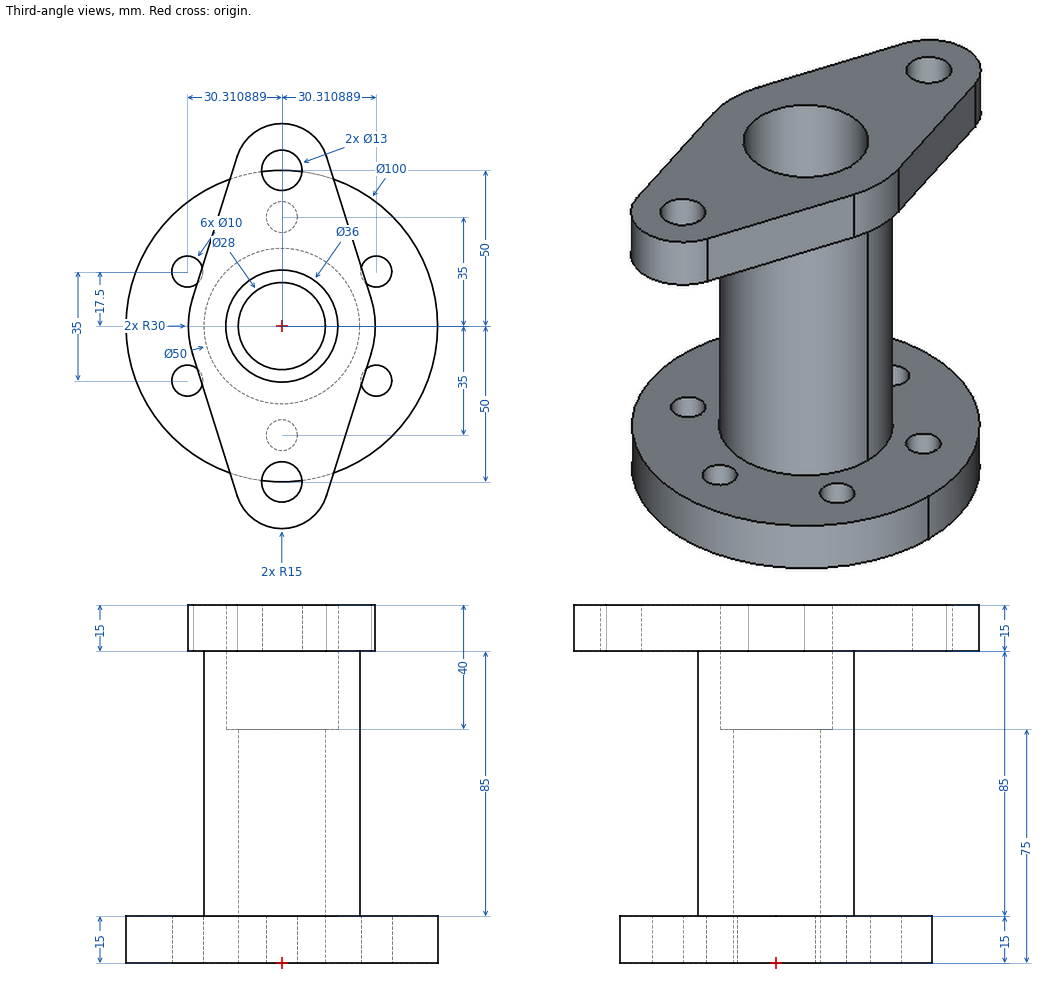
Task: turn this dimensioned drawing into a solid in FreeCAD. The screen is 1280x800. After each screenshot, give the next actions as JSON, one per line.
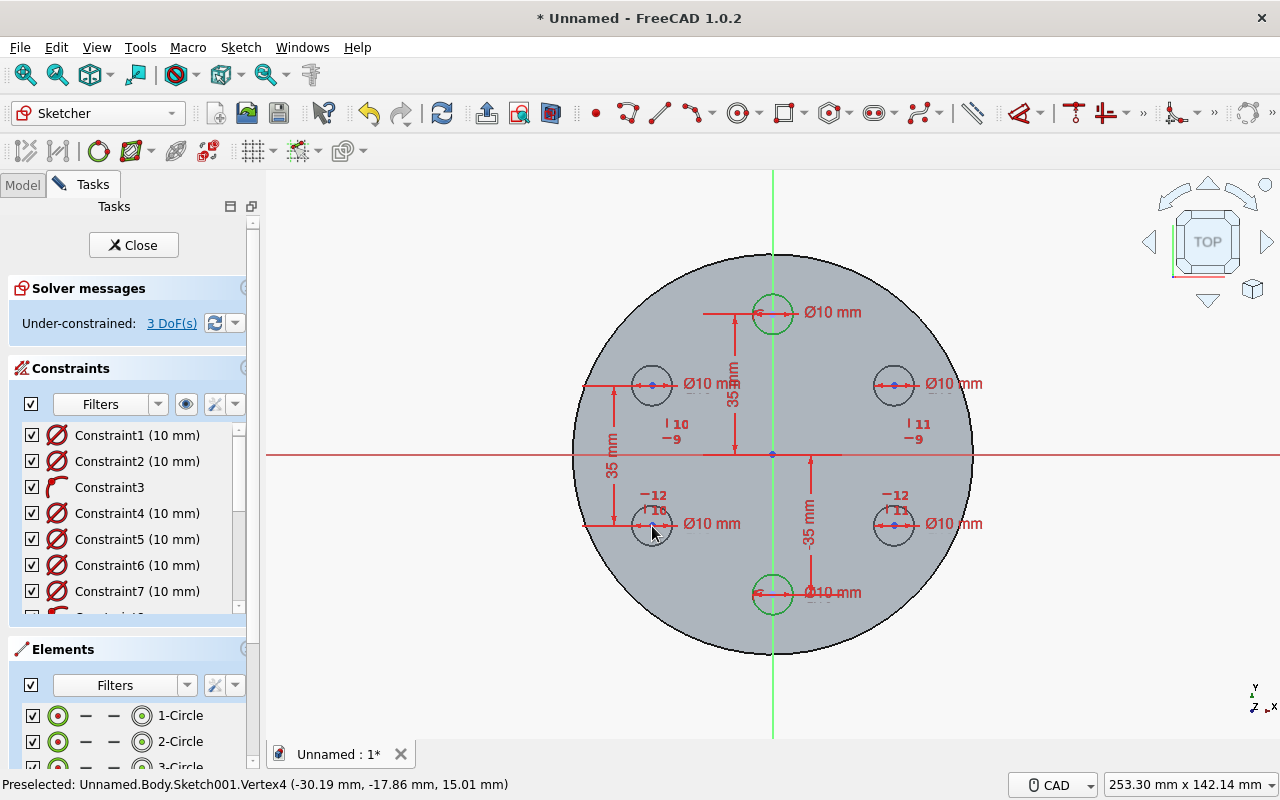
{"action": "left_click", "coordinate": [652, 386]}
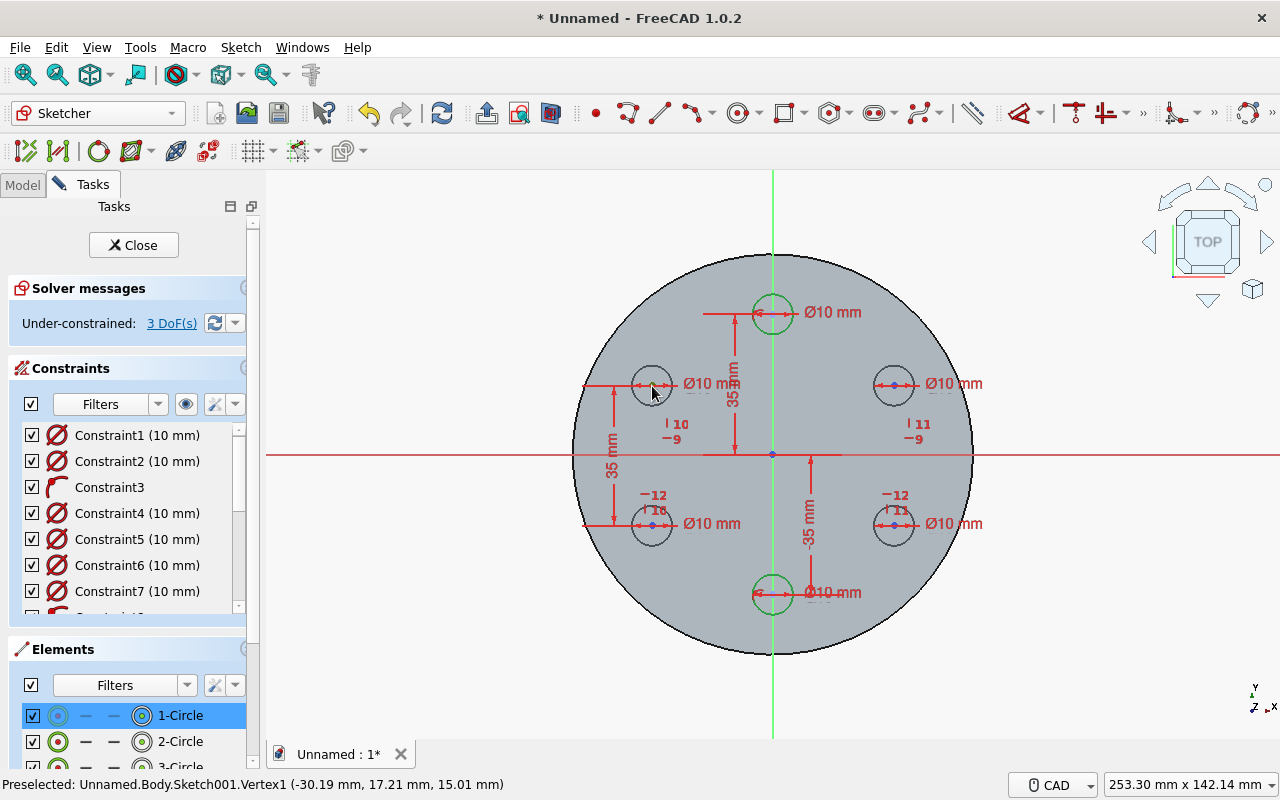
{"action": "key", "text": "i"}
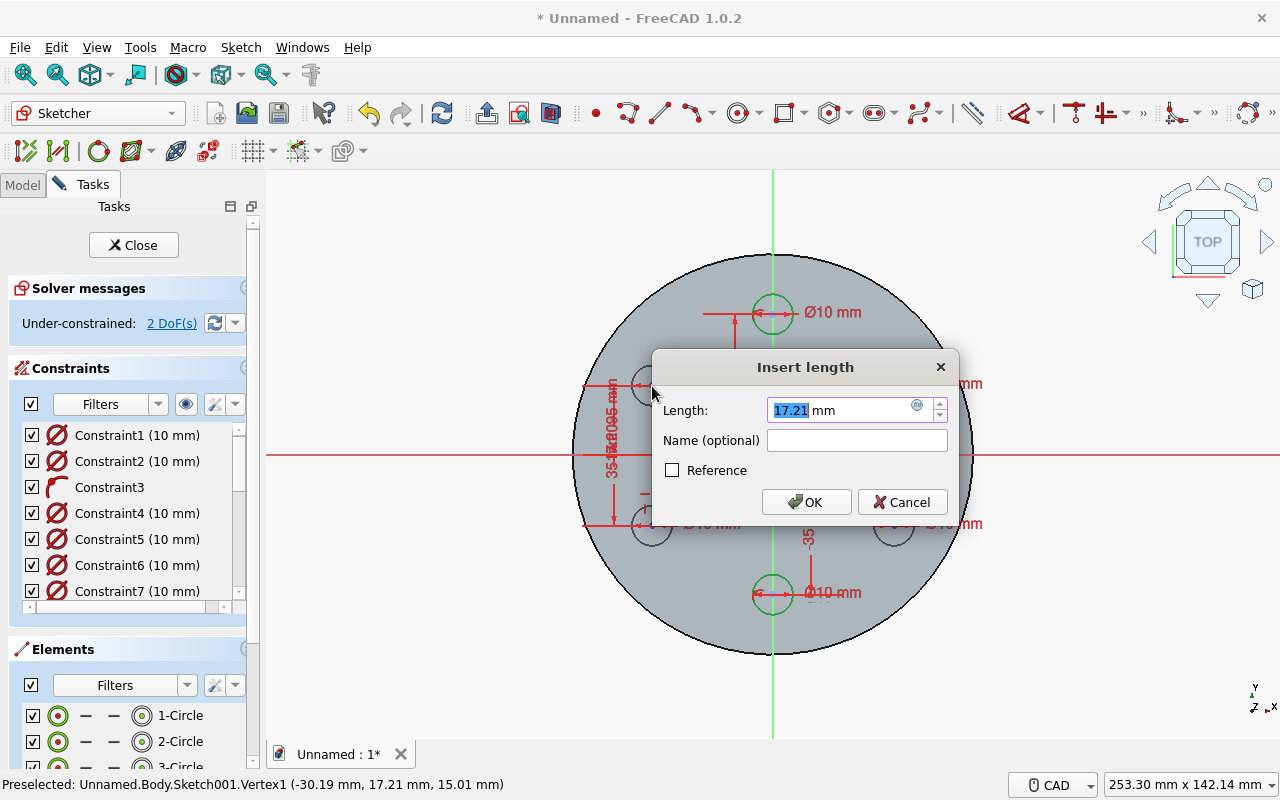
{"action": "type", "text": "17.5"}
{"action": "key", "text": "Return"}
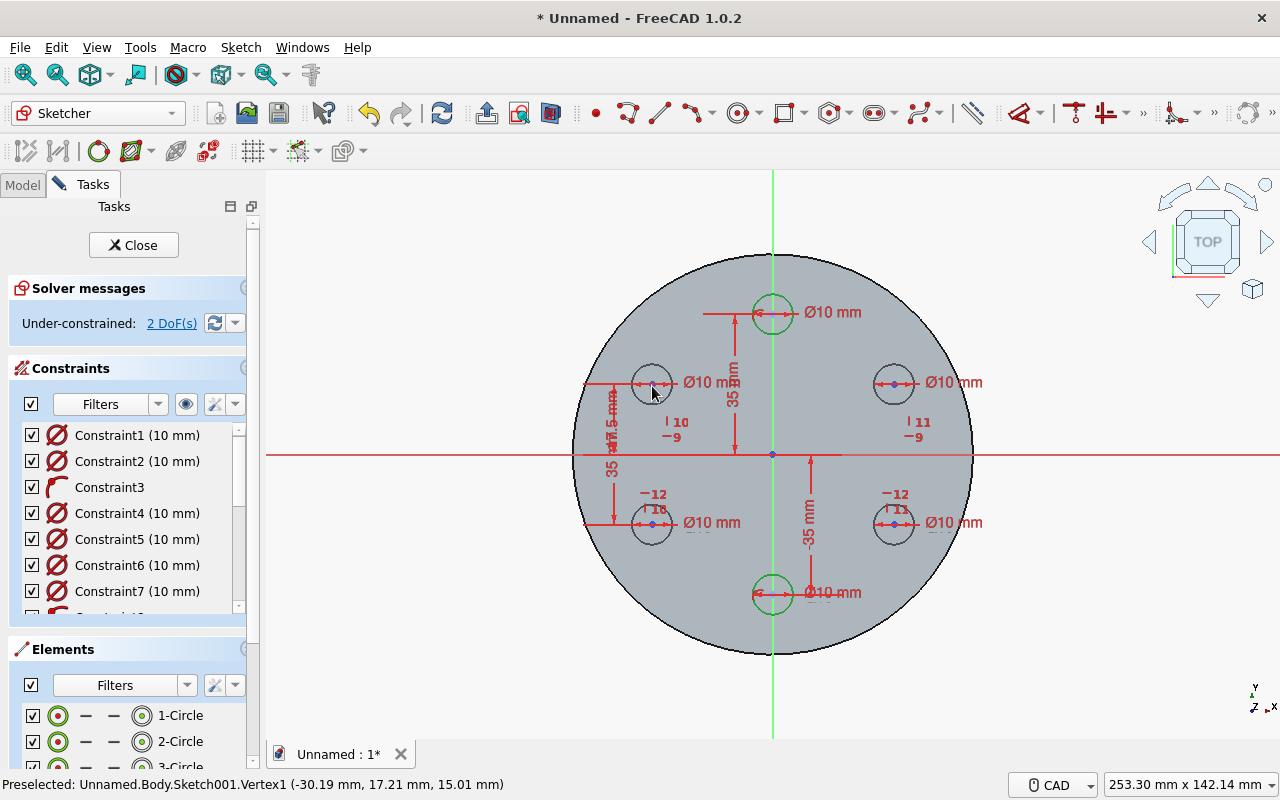
{"action": "left_click", "coordinate": [652, 384]}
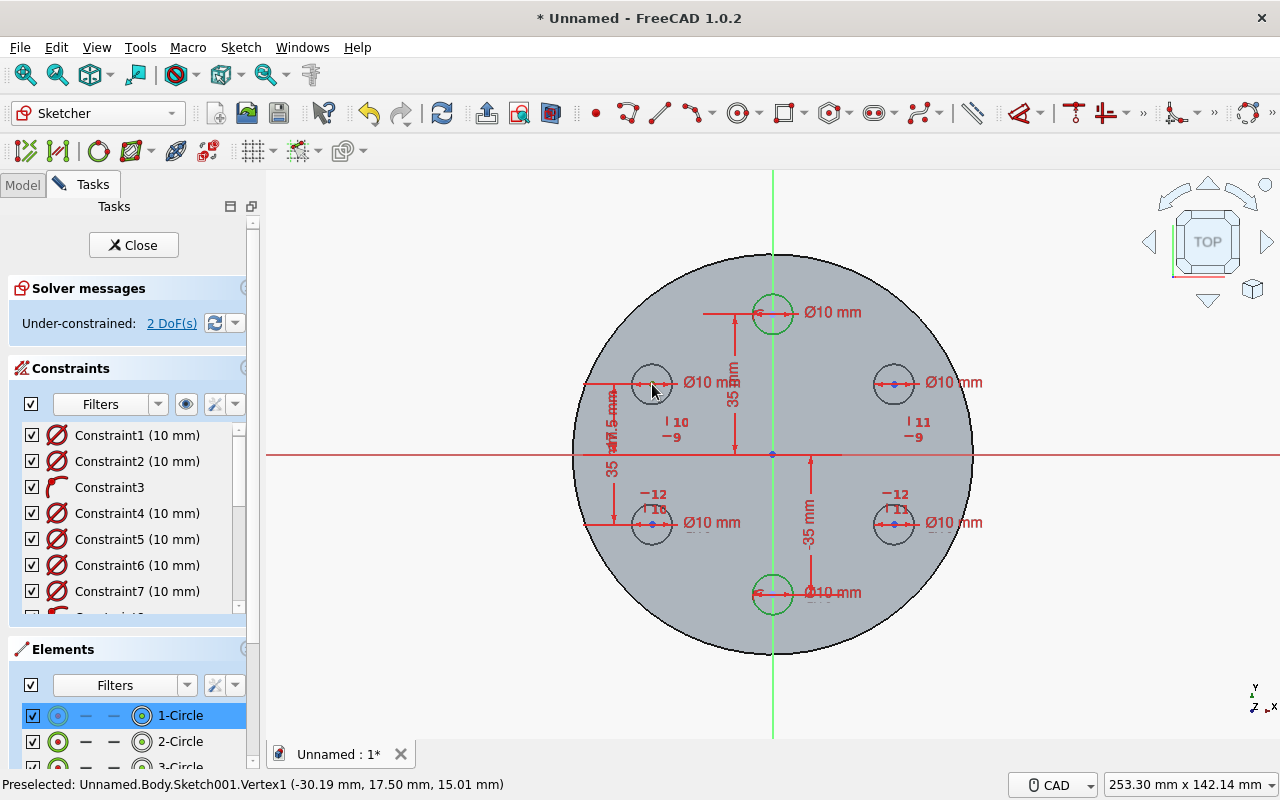
{"action": "key", "text": "l"}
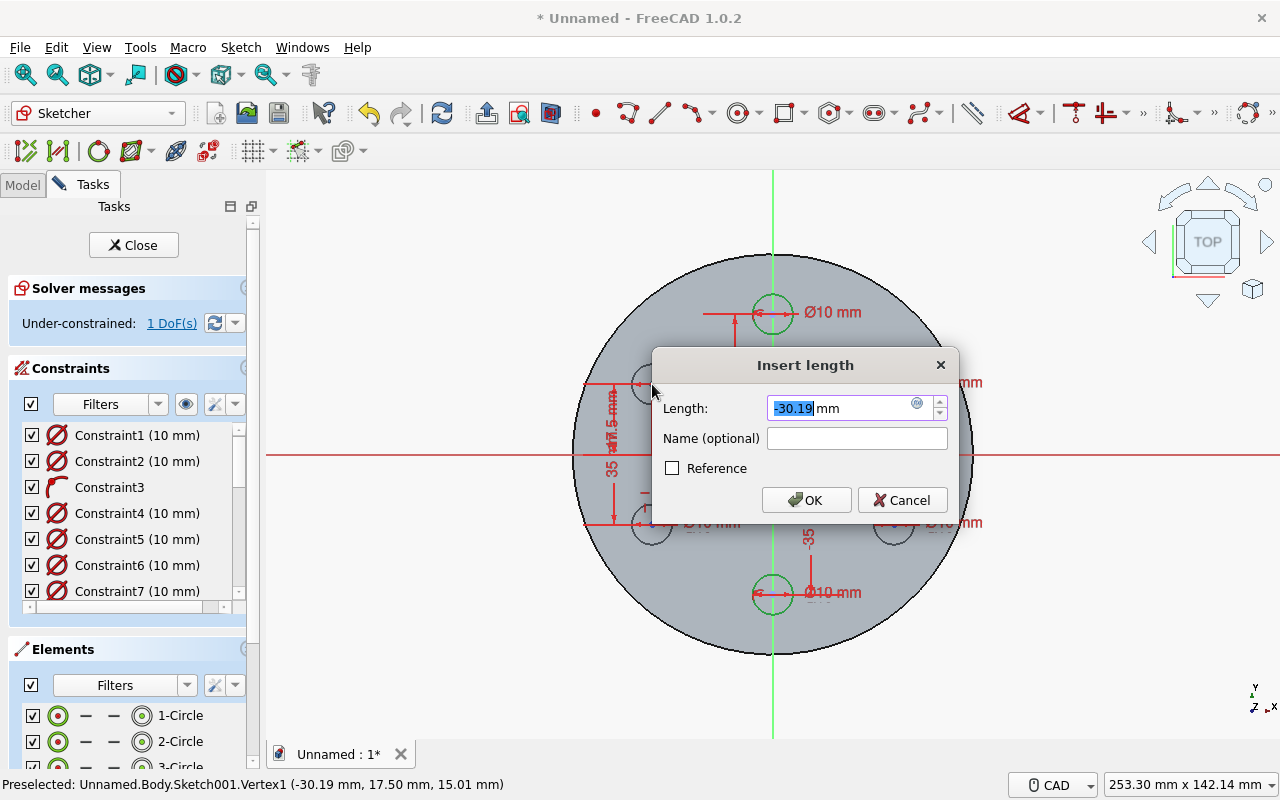
{"action": "type", "text": "-30.310889"}
{"action": "key", "text": "Return"}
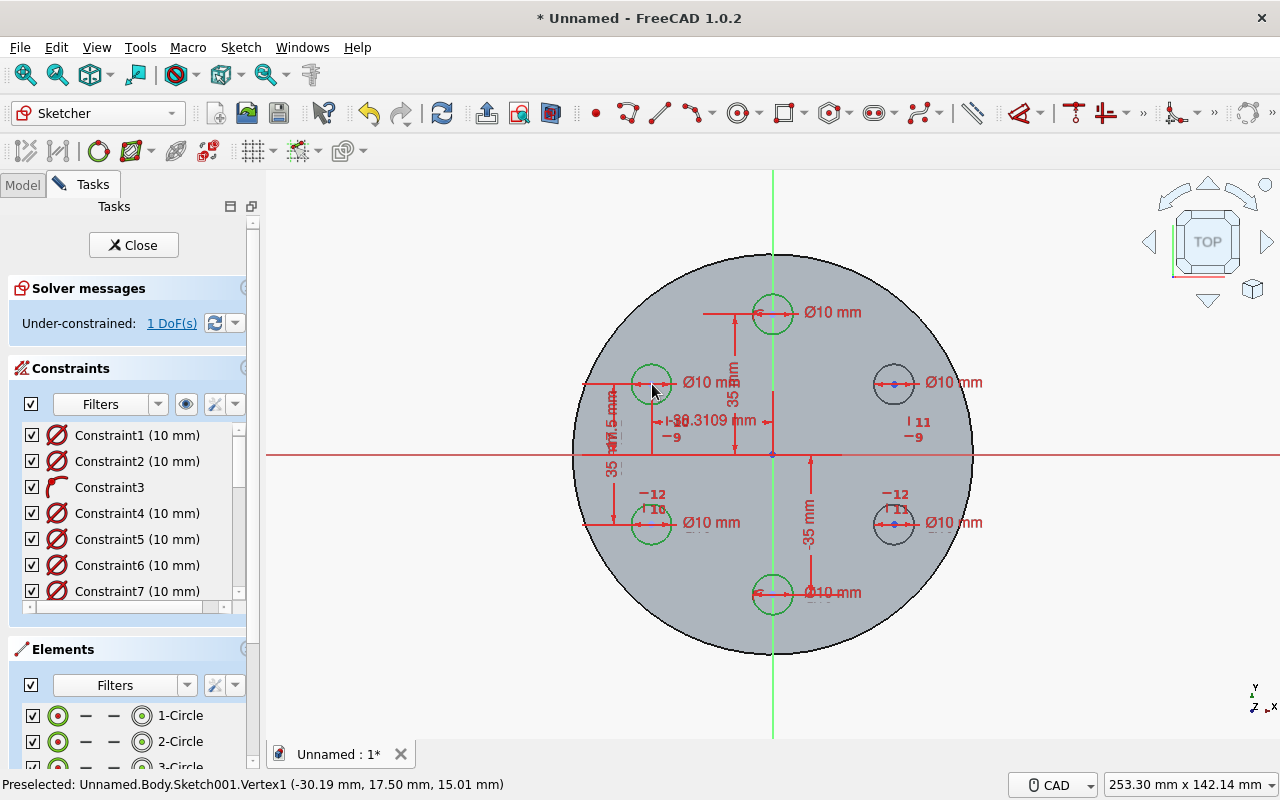
{"action": "left_click", "coordinate": [894, 384]}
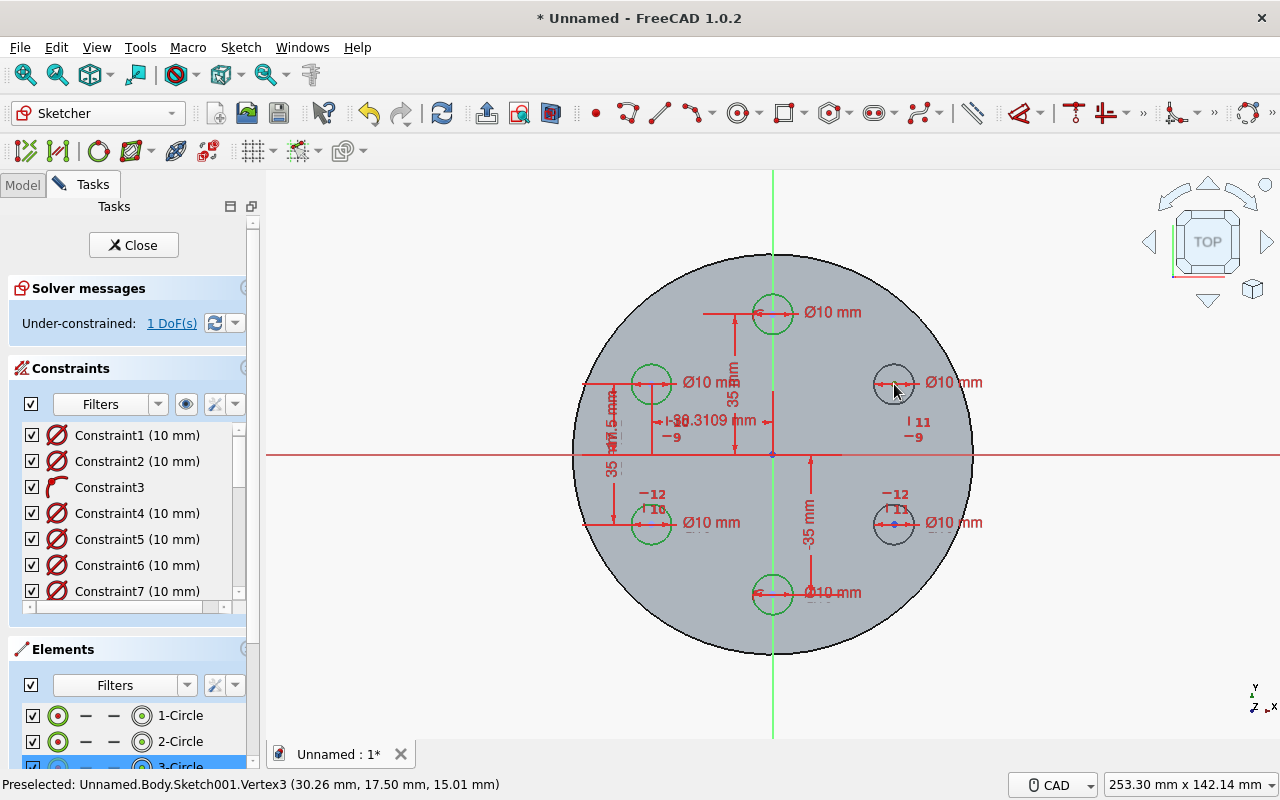
{"action": "key", "text": "l"}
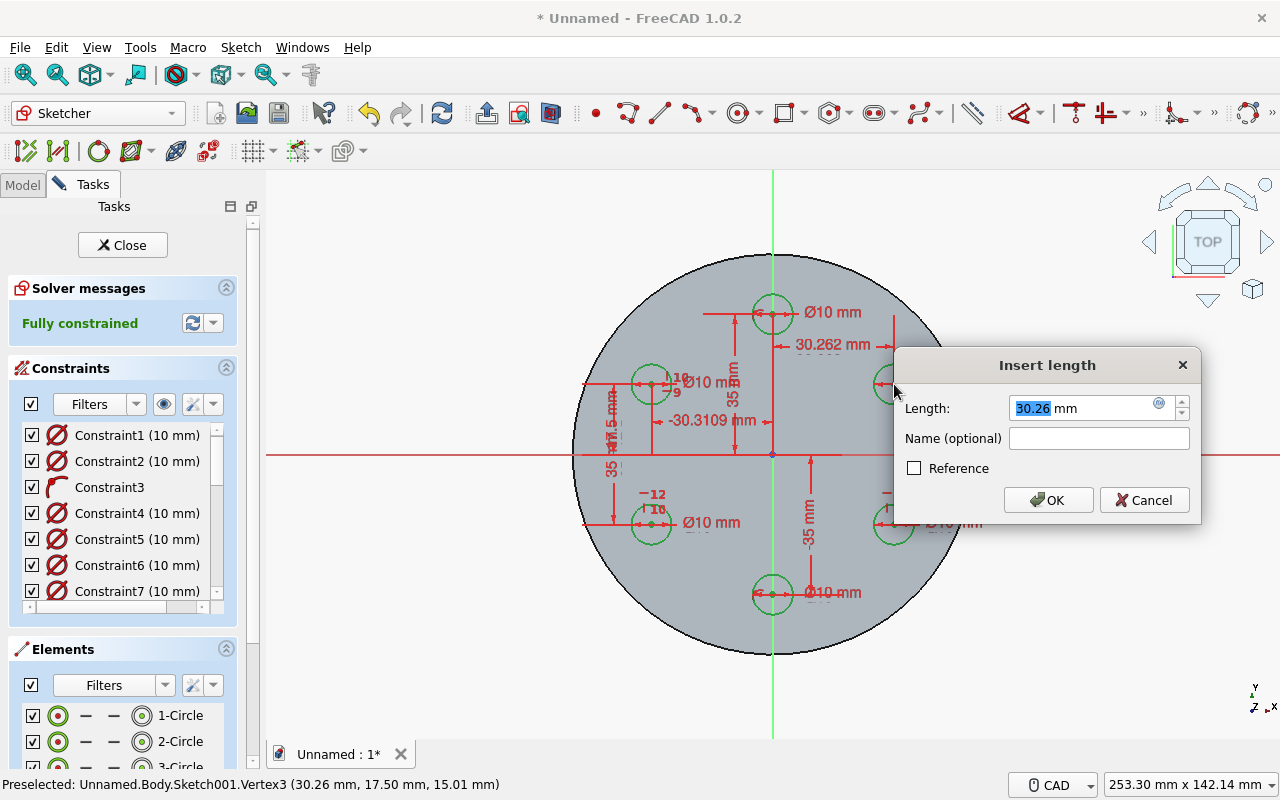
{"action": "type", "text": "30.310889"}
{"action": "key", "text": "Return"}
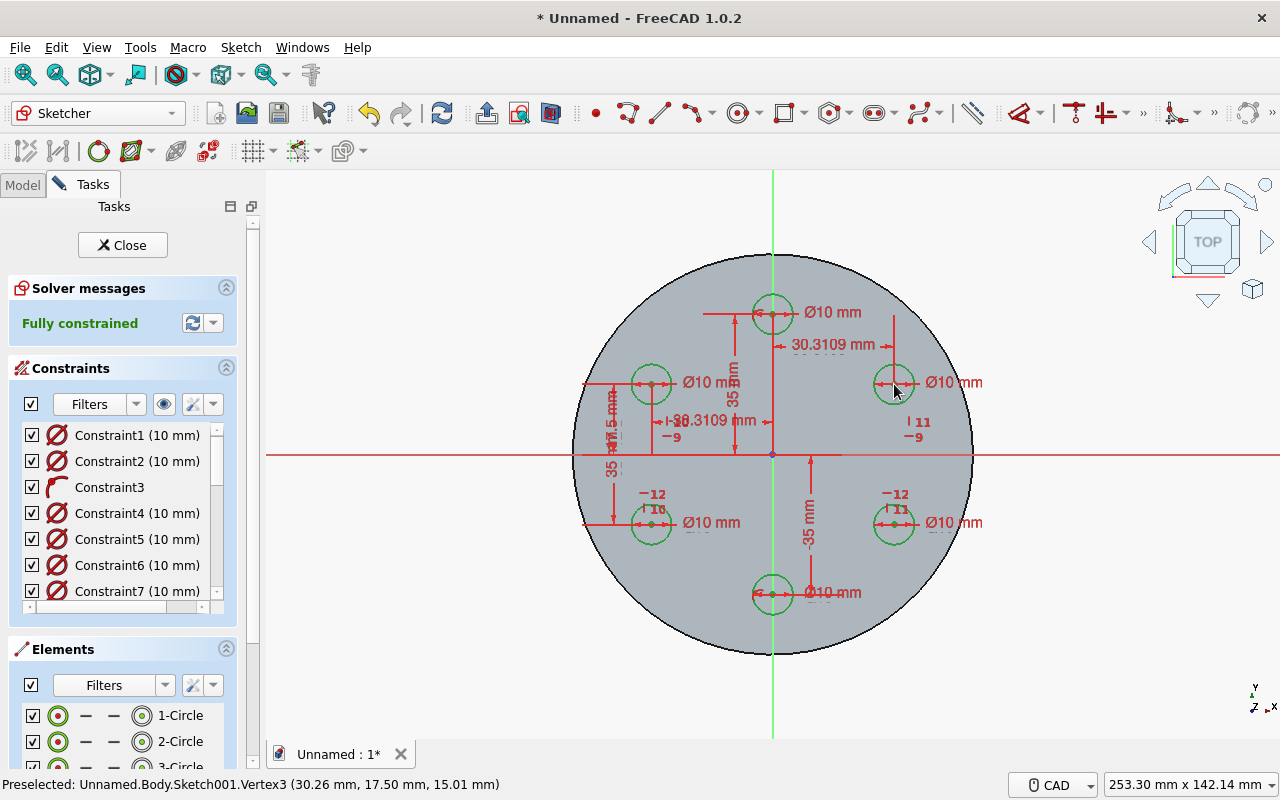
{"action": "left_click", "coordinate": [123, 245]}